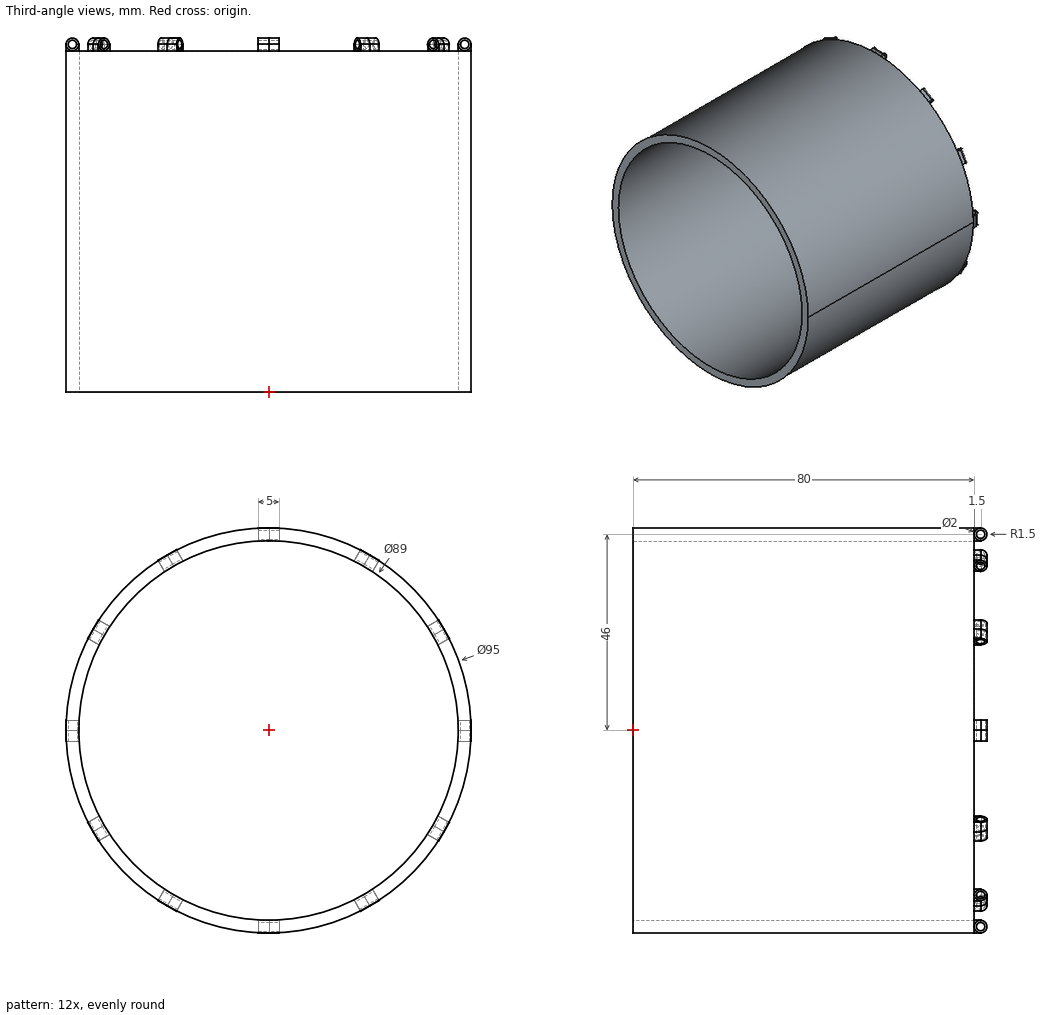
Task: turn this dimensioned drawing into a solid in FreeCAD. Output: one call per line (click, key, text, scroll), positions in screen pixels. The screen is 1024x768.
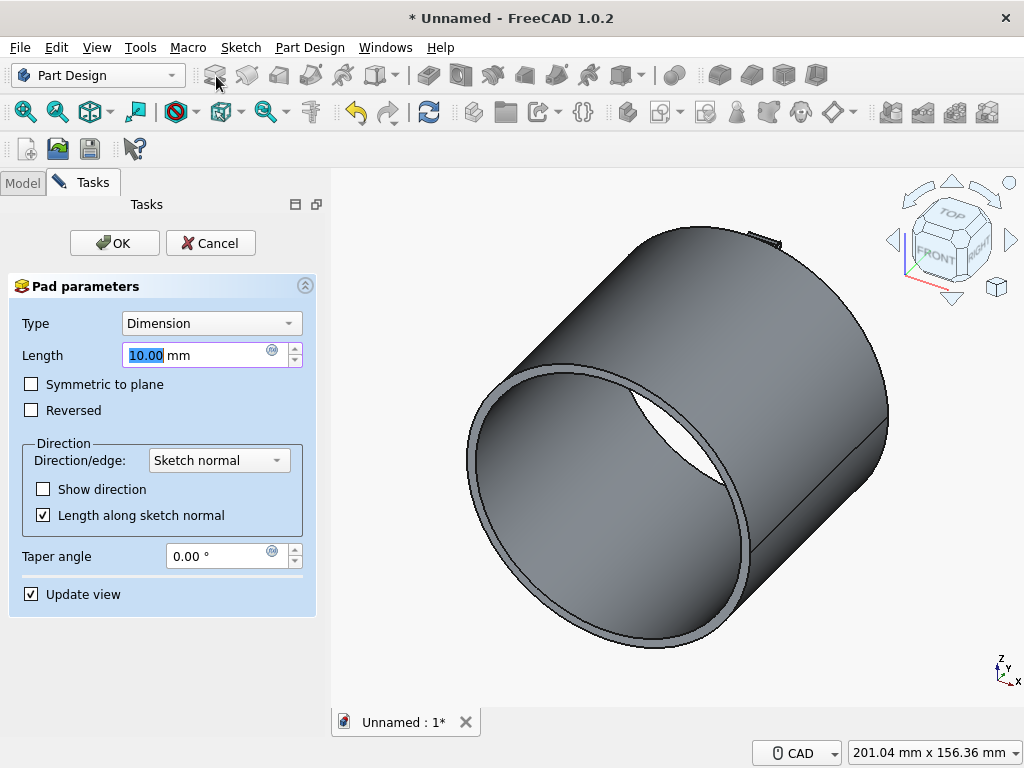
text(5)
key(Tab)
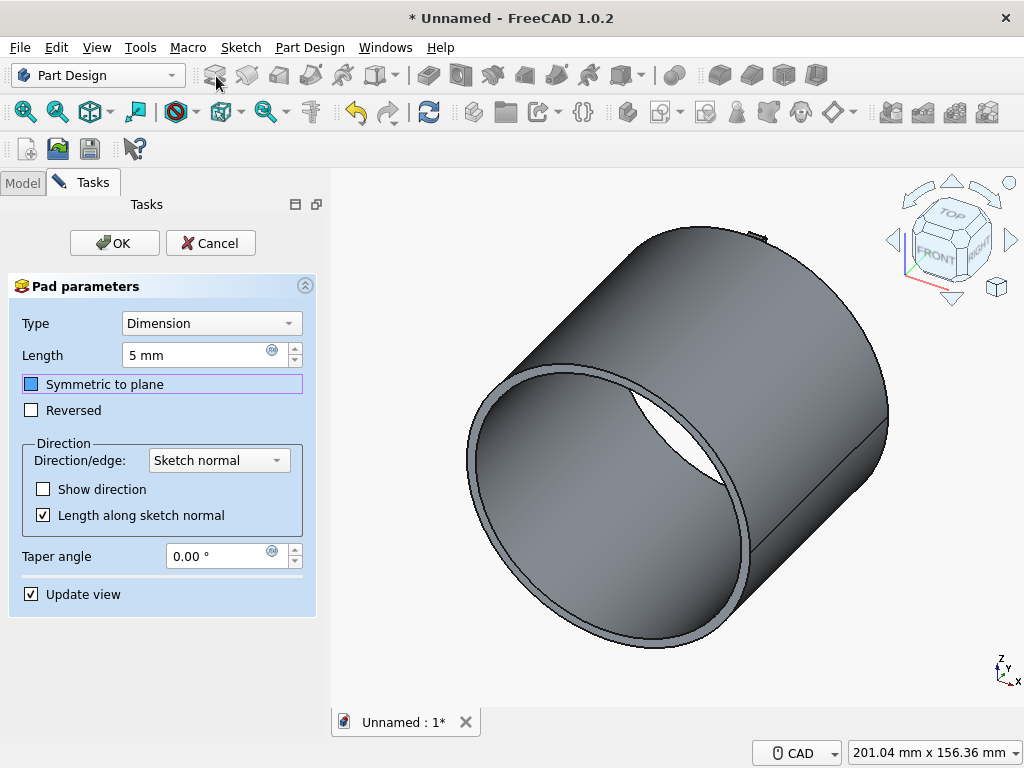
click(30, 384)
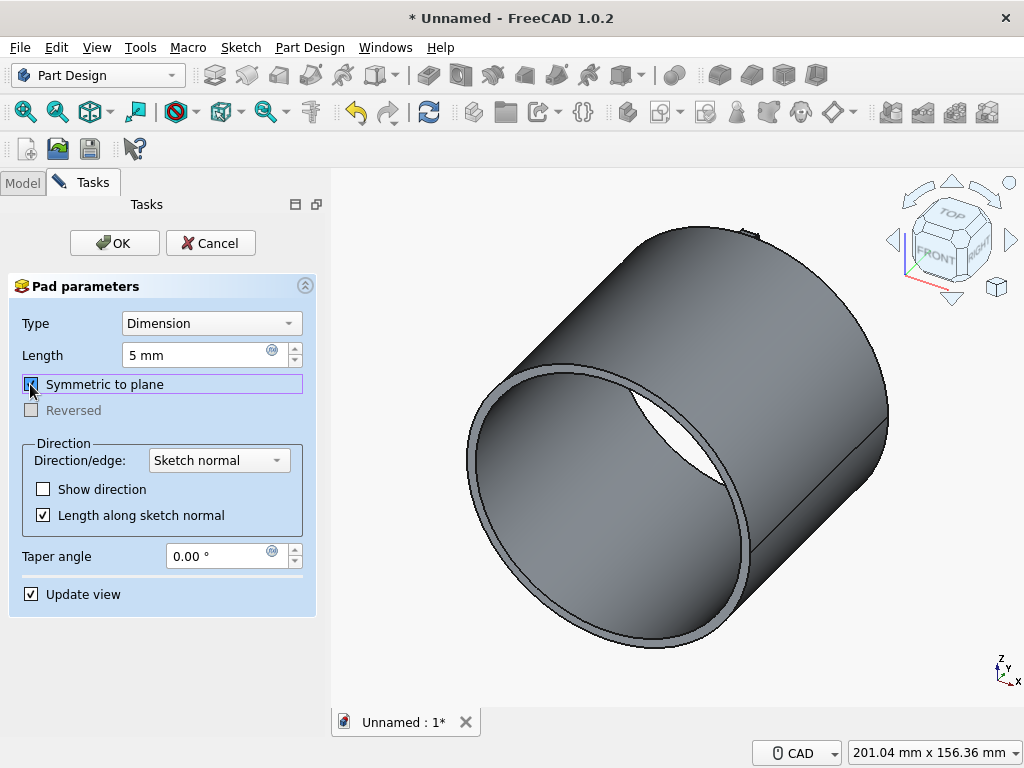
click(115, 243)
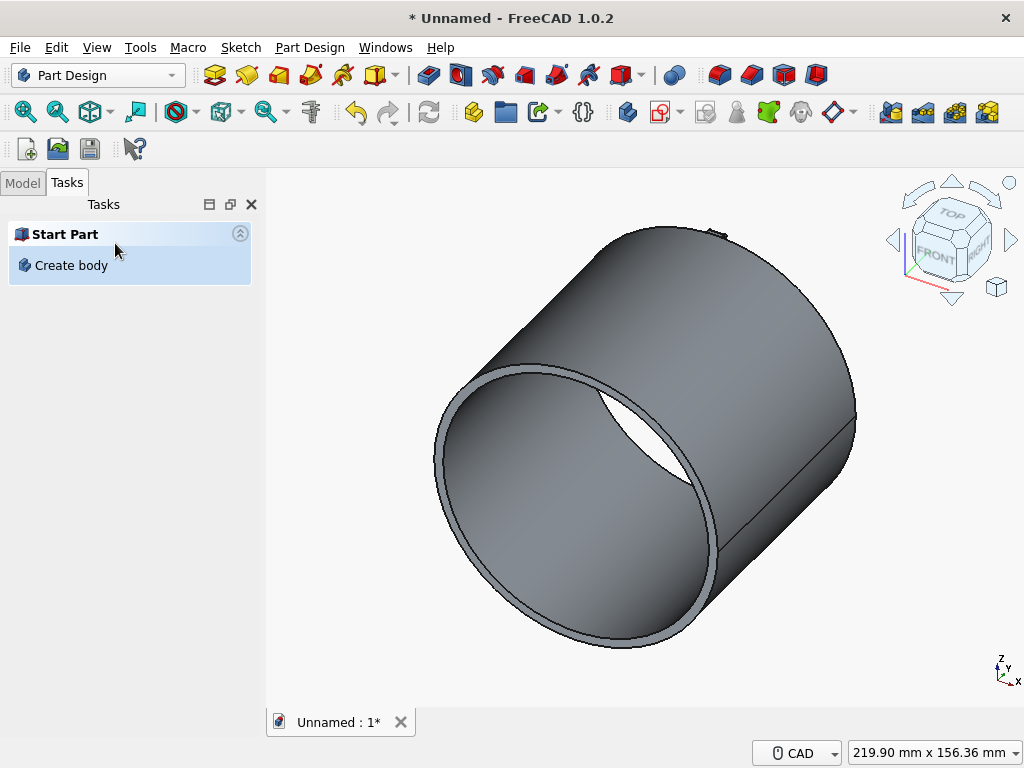
click(23, 182)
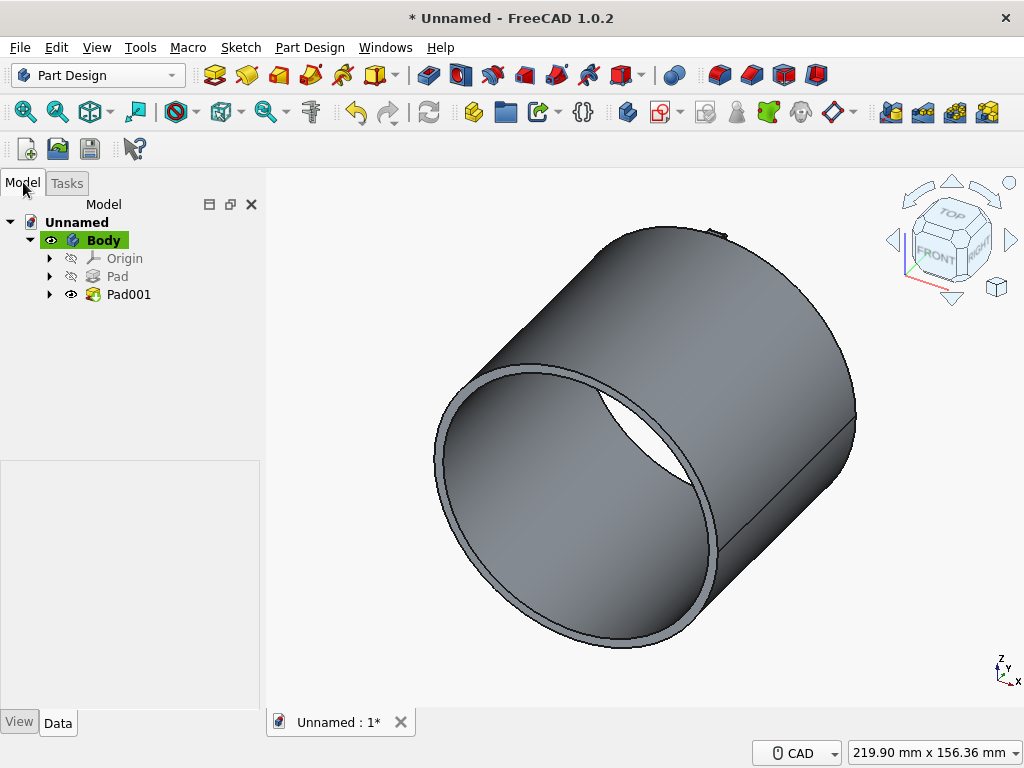
click(116, 294)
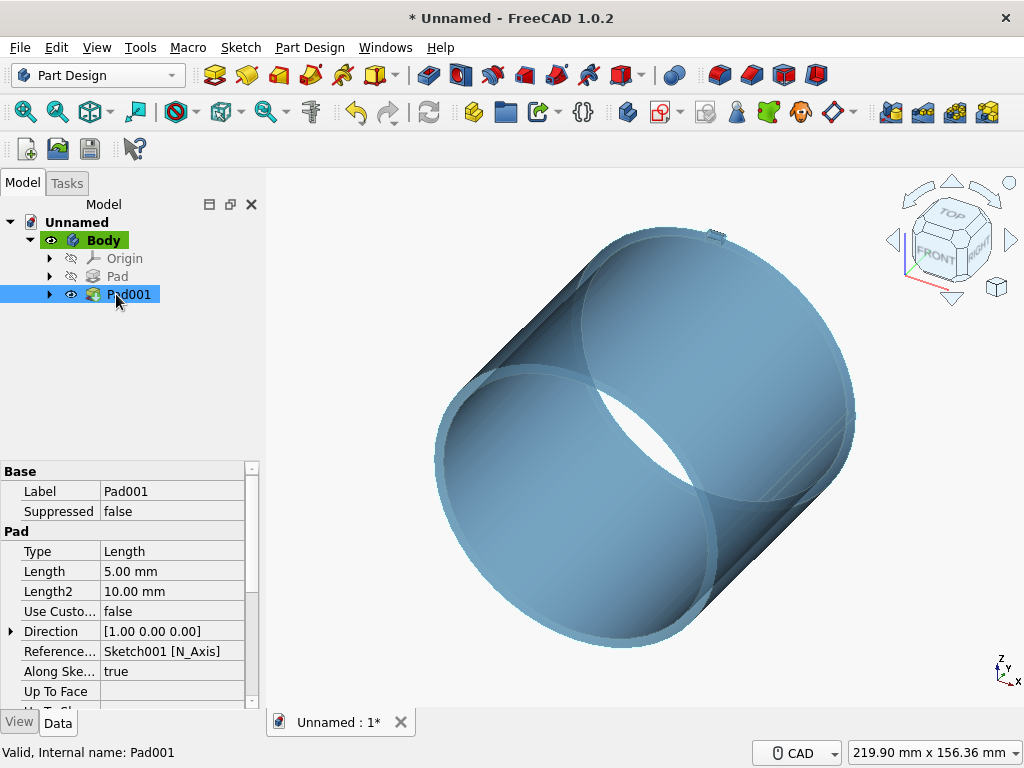
click(956, 112)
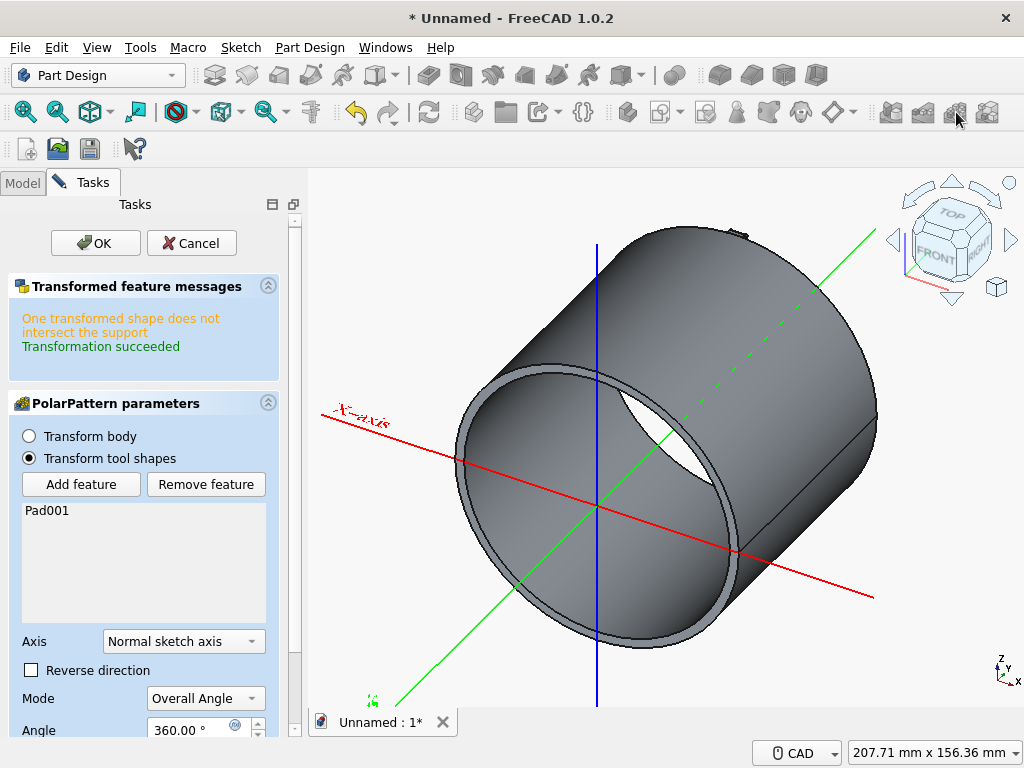
click(184, 642)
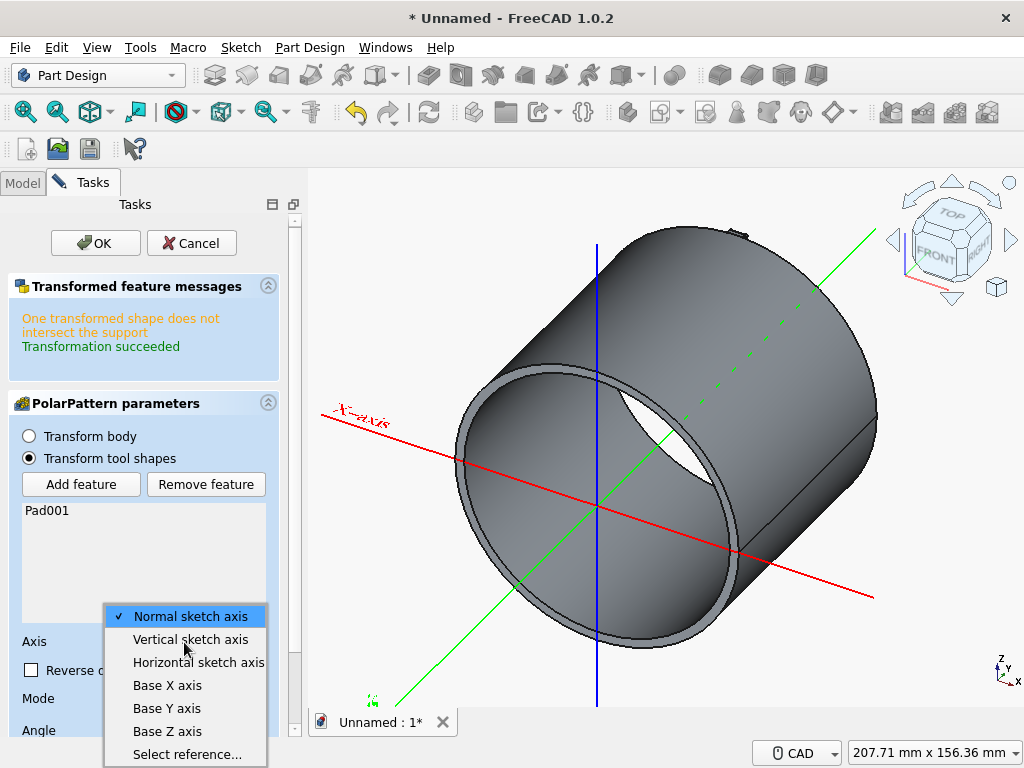
click(184, 708)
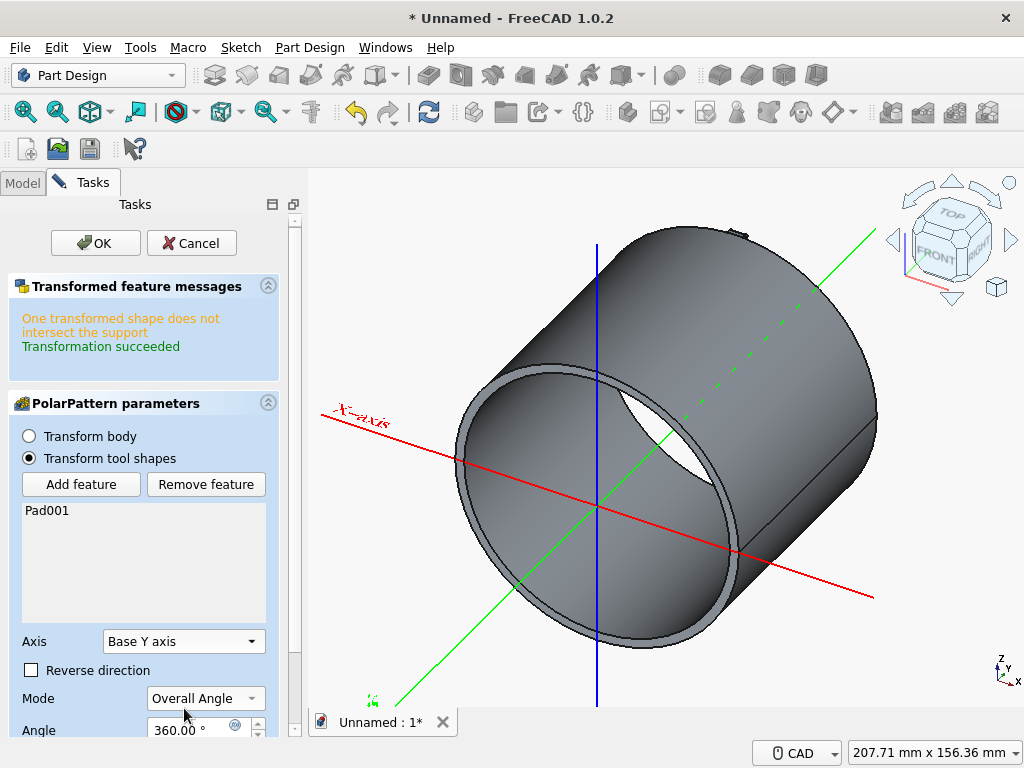
scroll(295, 475, down, 2)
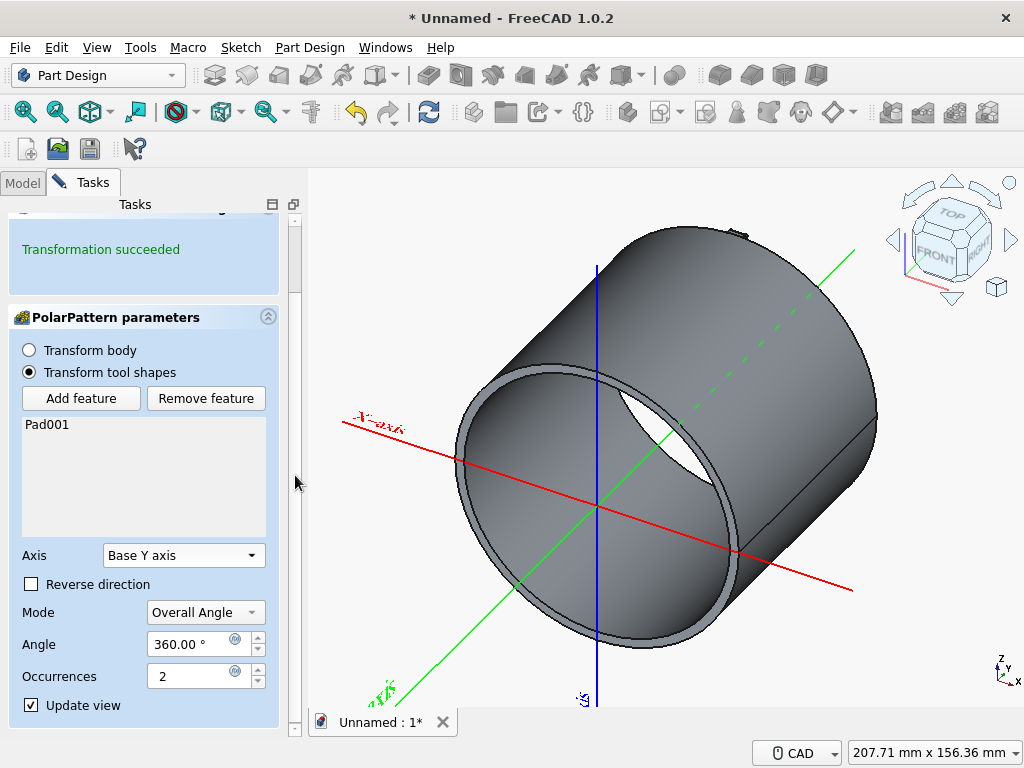
triple_click(198, 676)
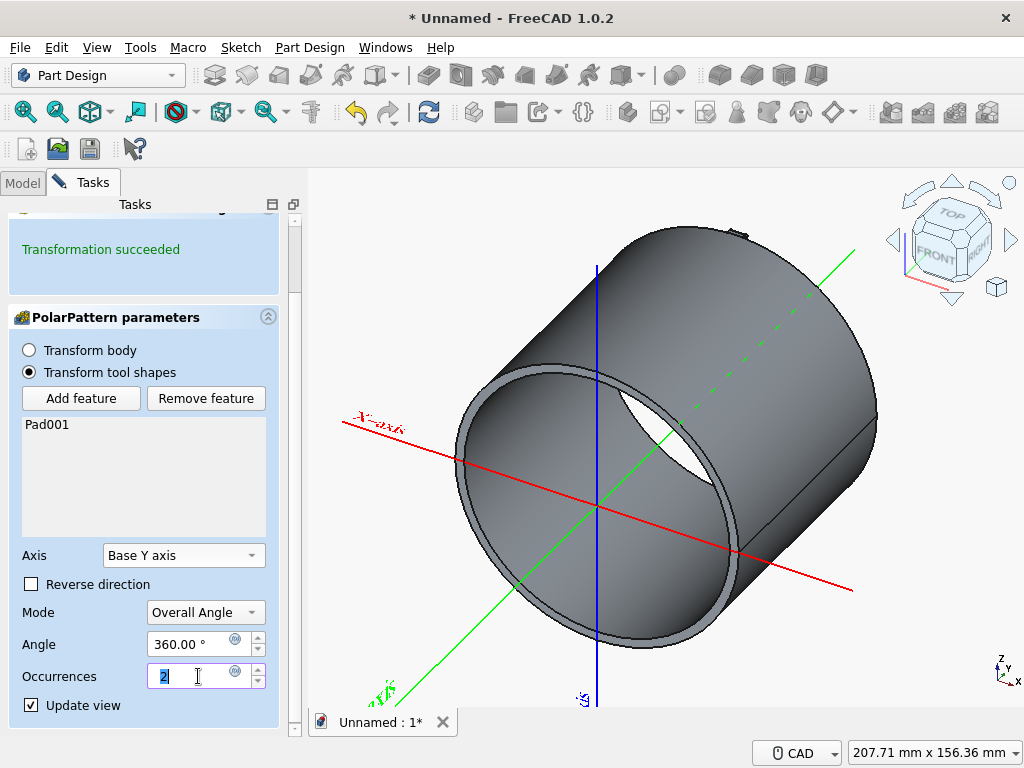
text(12)
key(Tab)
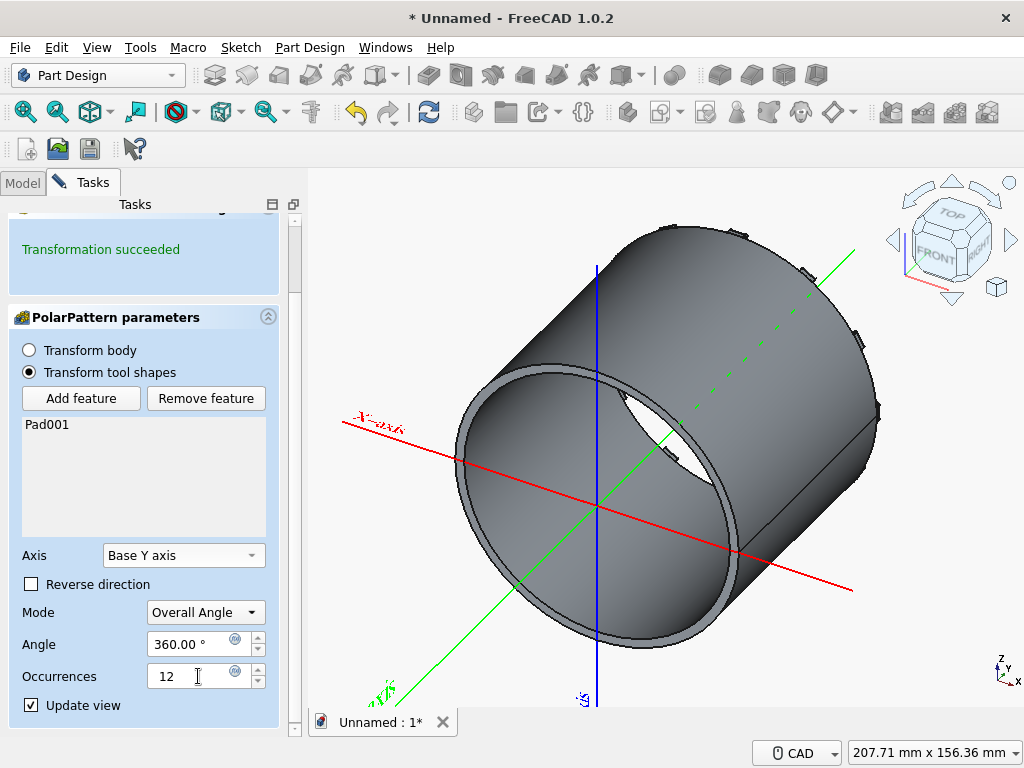
scroll(295, 475, up, 3)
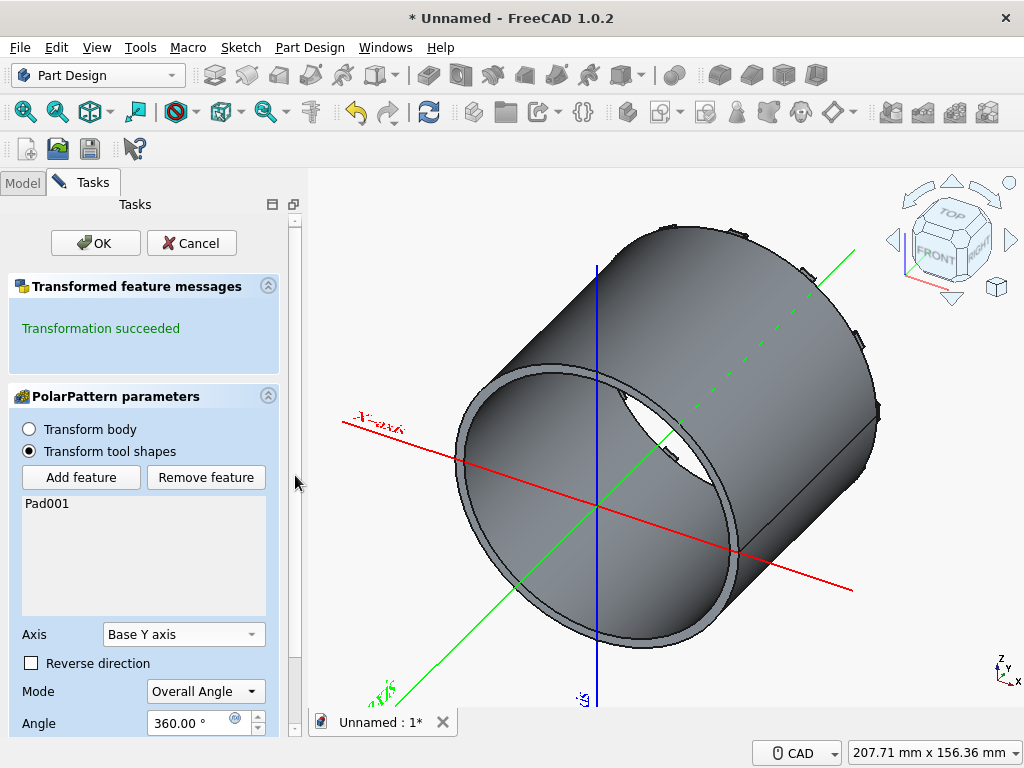
click(96, 243)